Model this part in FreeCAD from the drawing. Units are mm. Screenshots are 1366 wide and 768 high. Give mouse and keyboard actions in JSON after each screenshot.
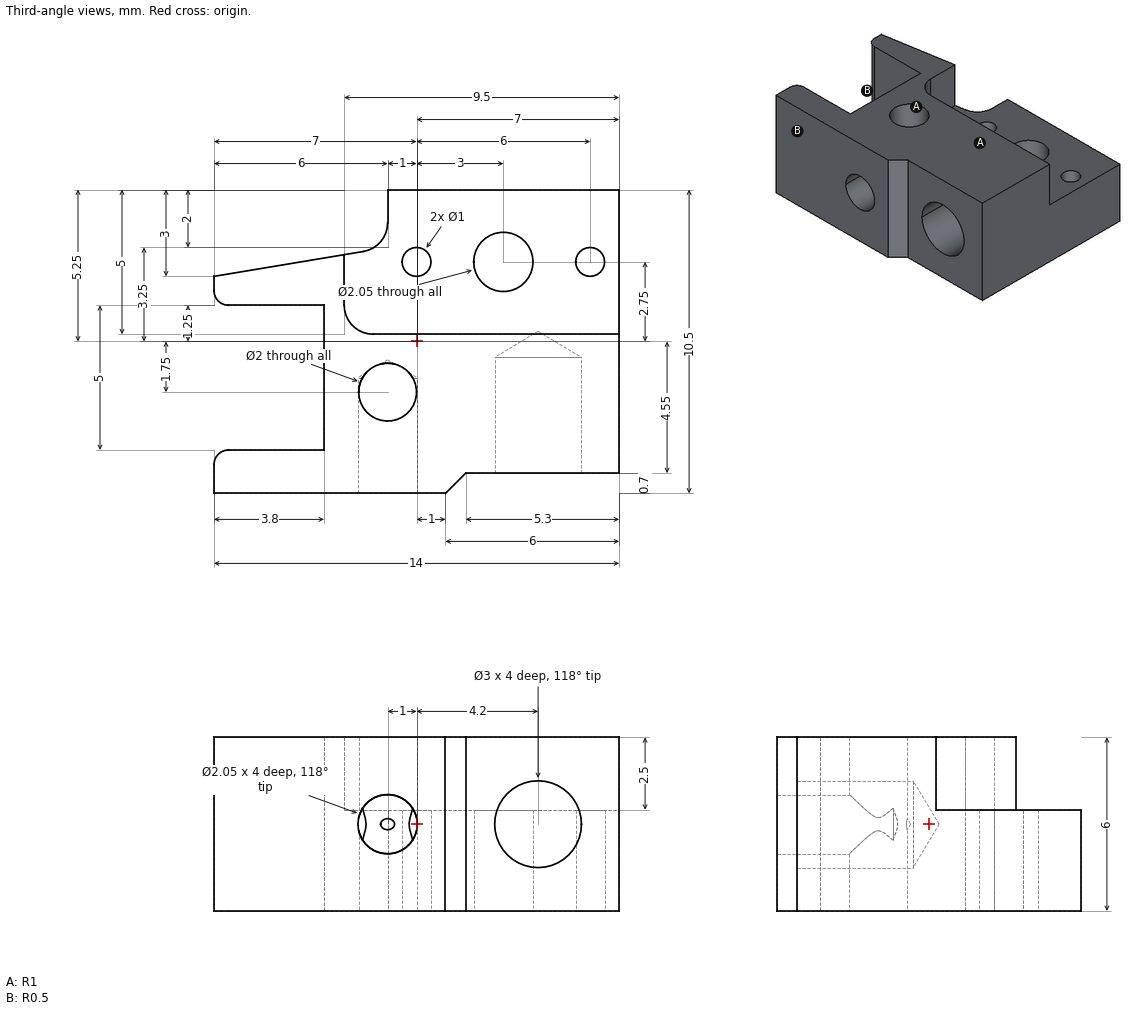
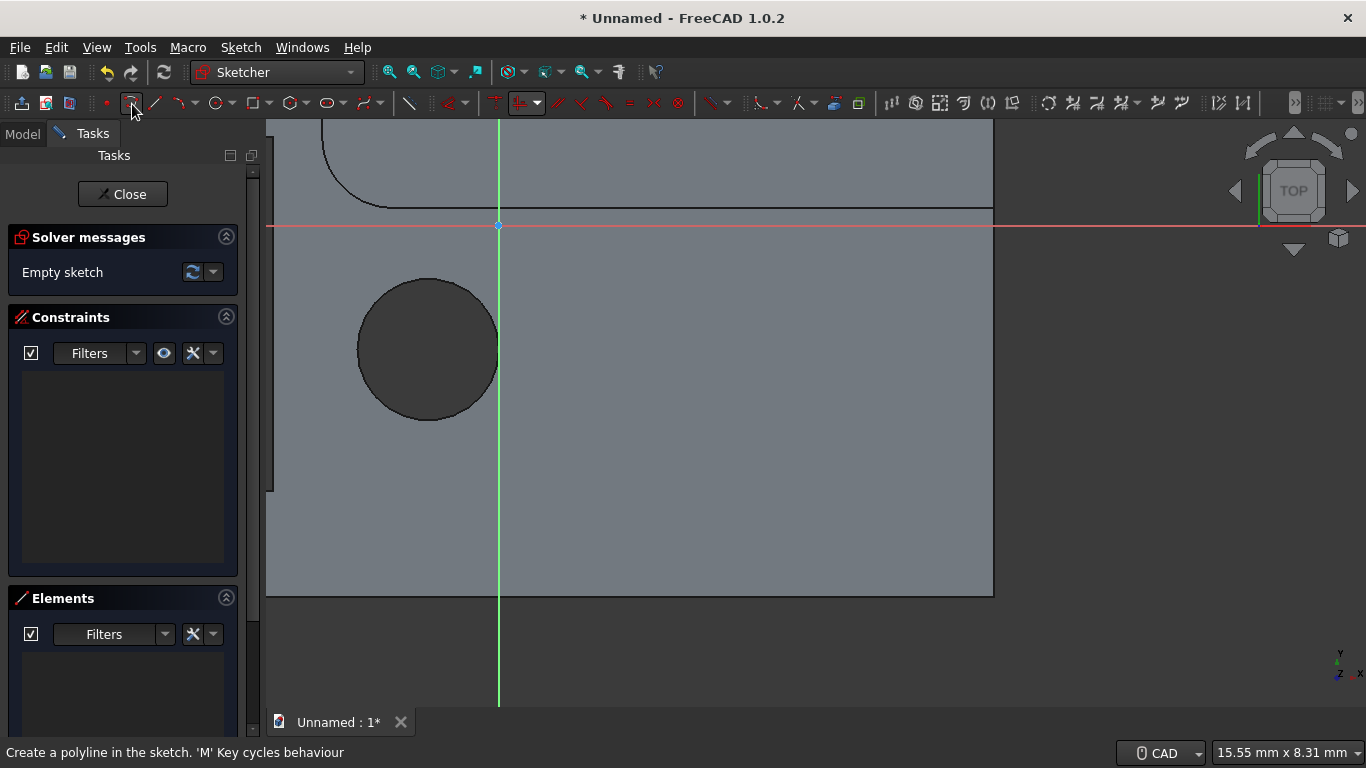
{"action": "left_click", "coordinate": [619, 548]}
{"action": "left_click", "coordinate": [570, 597]}
{"action": "left_click", "coordinate": [994, 597]}
{"action": "left_click", "coordinate": [994, 548]}
{"action": "left_click", "coordinate": [619, 549]}
{"action": "key", "text": "Escape"}
{"action": "key", "text": "Escape"}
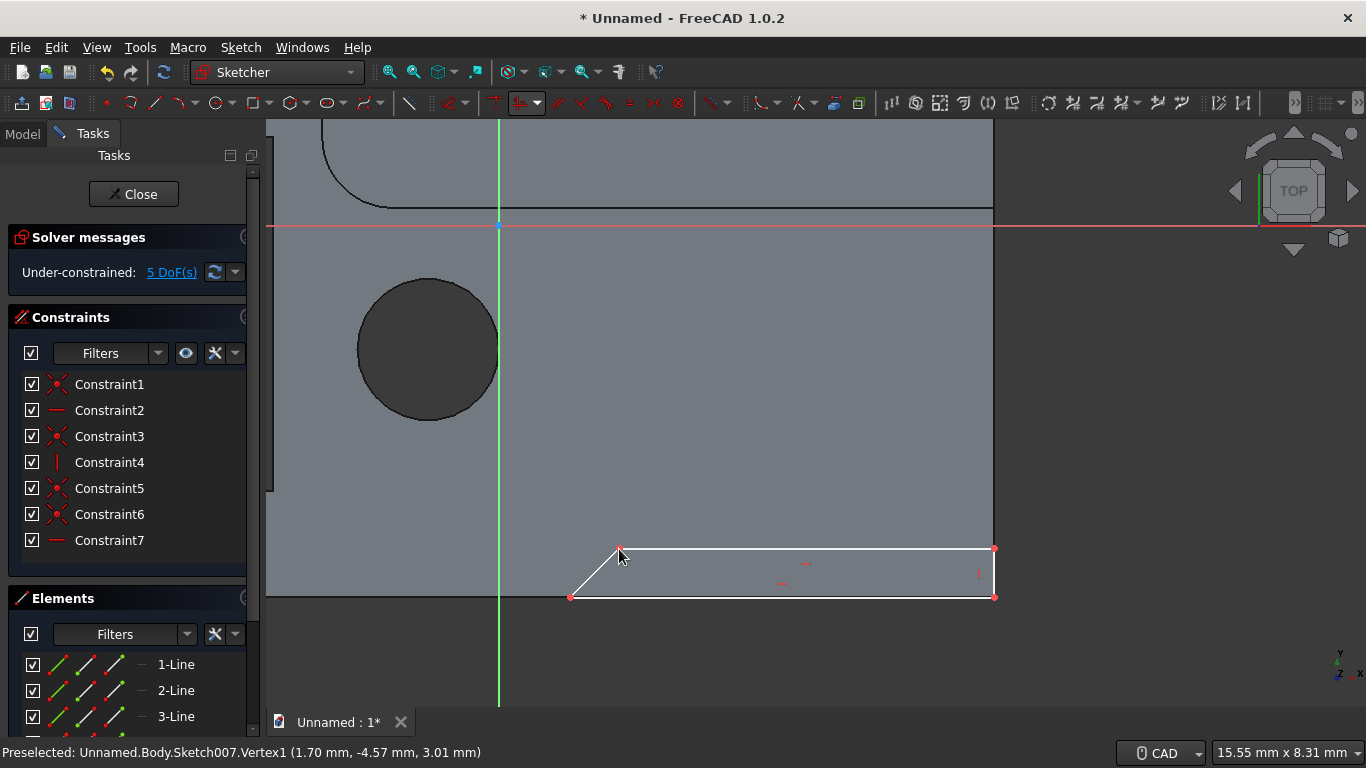
{"action": "left_click", "coordinate": [448, 104]}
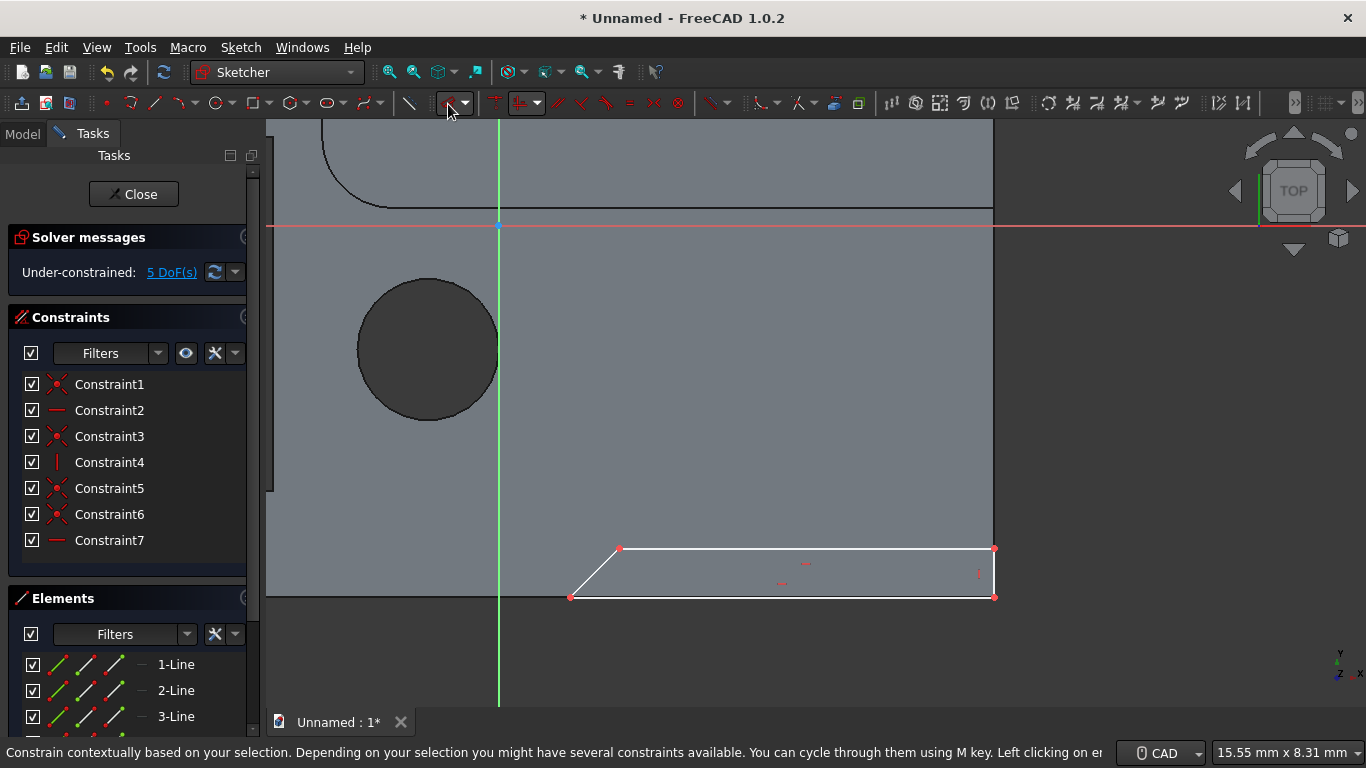
{"action": "left_click", "coordinate": [697, 598]}
{"action": "left_click", "coordinate": [782, 632]}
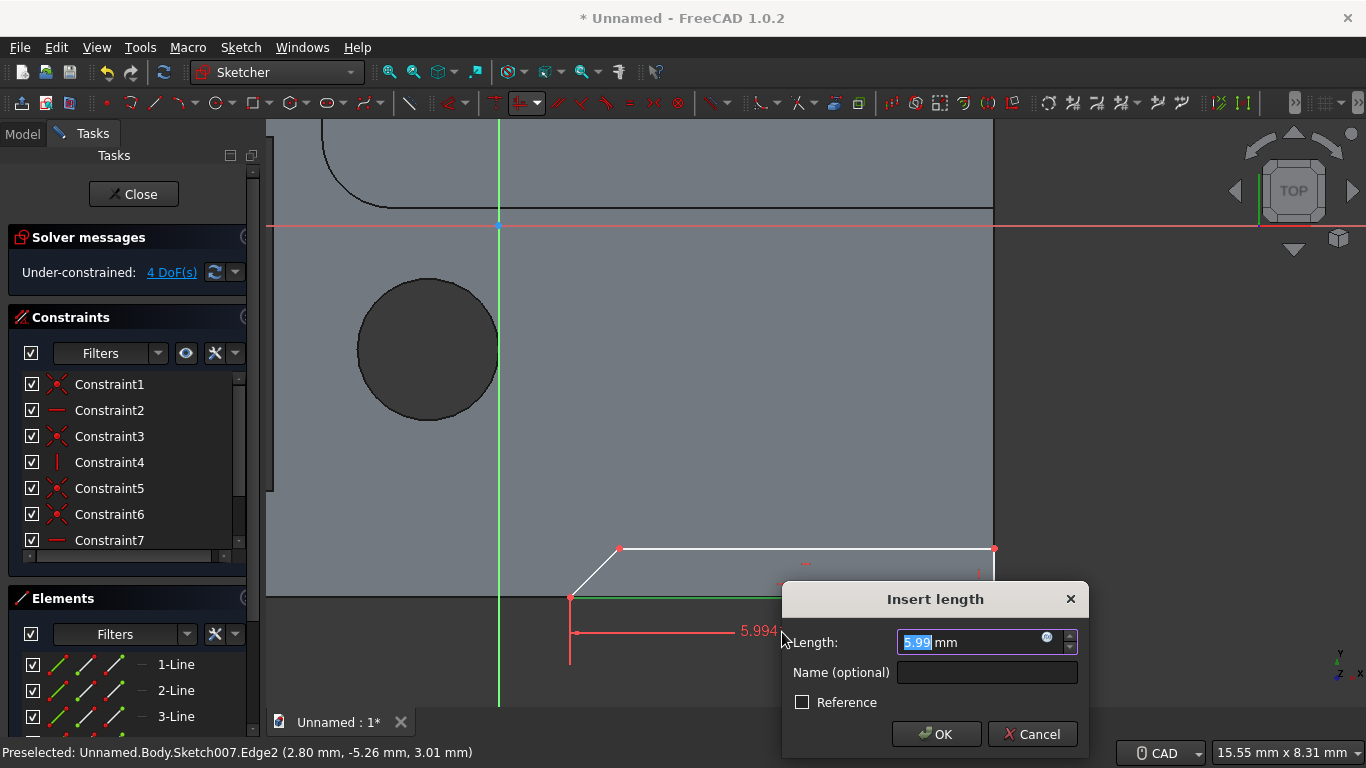
{"action": "type", "text": "6"}
{"action": "key", "text": "Return"}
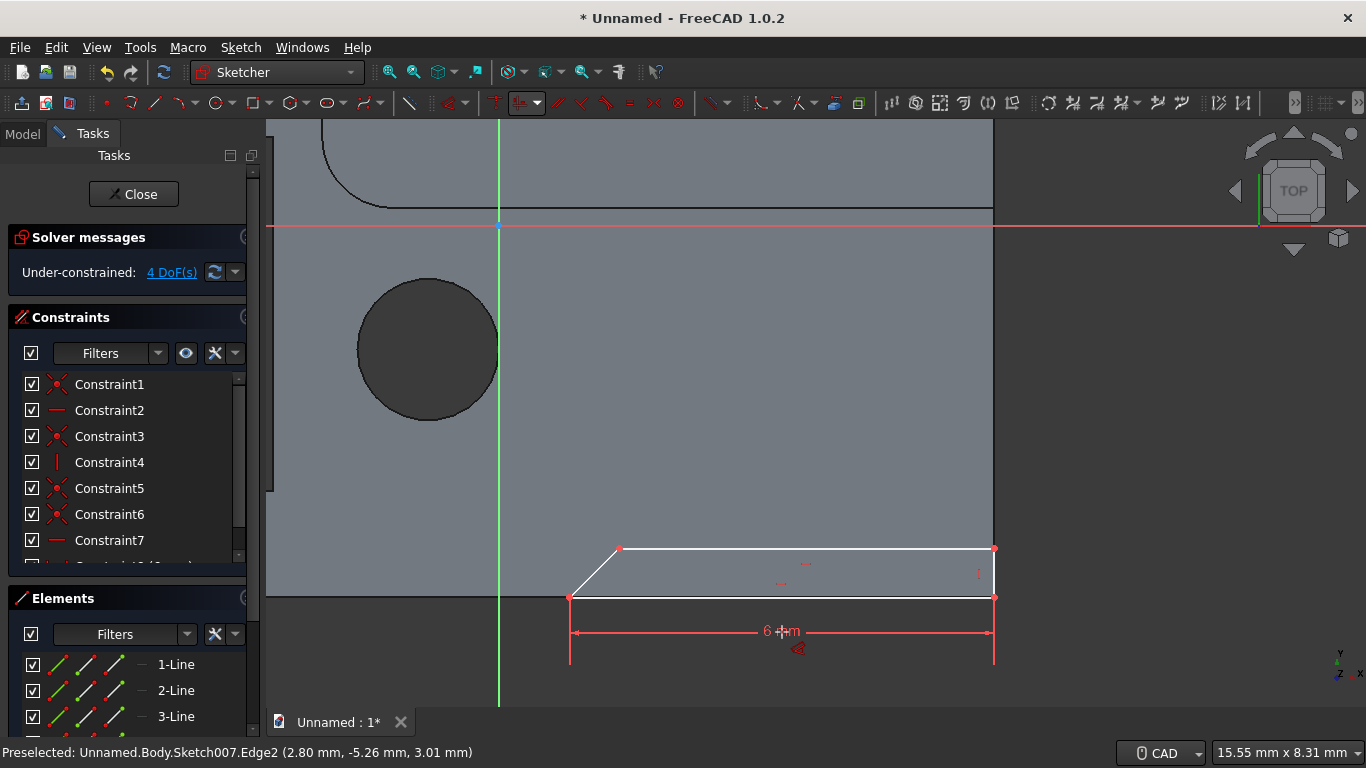
{"action": "left_click", "coordinate": [570, 598]}
{"action": "left_click", "coordinate": [534, 632]}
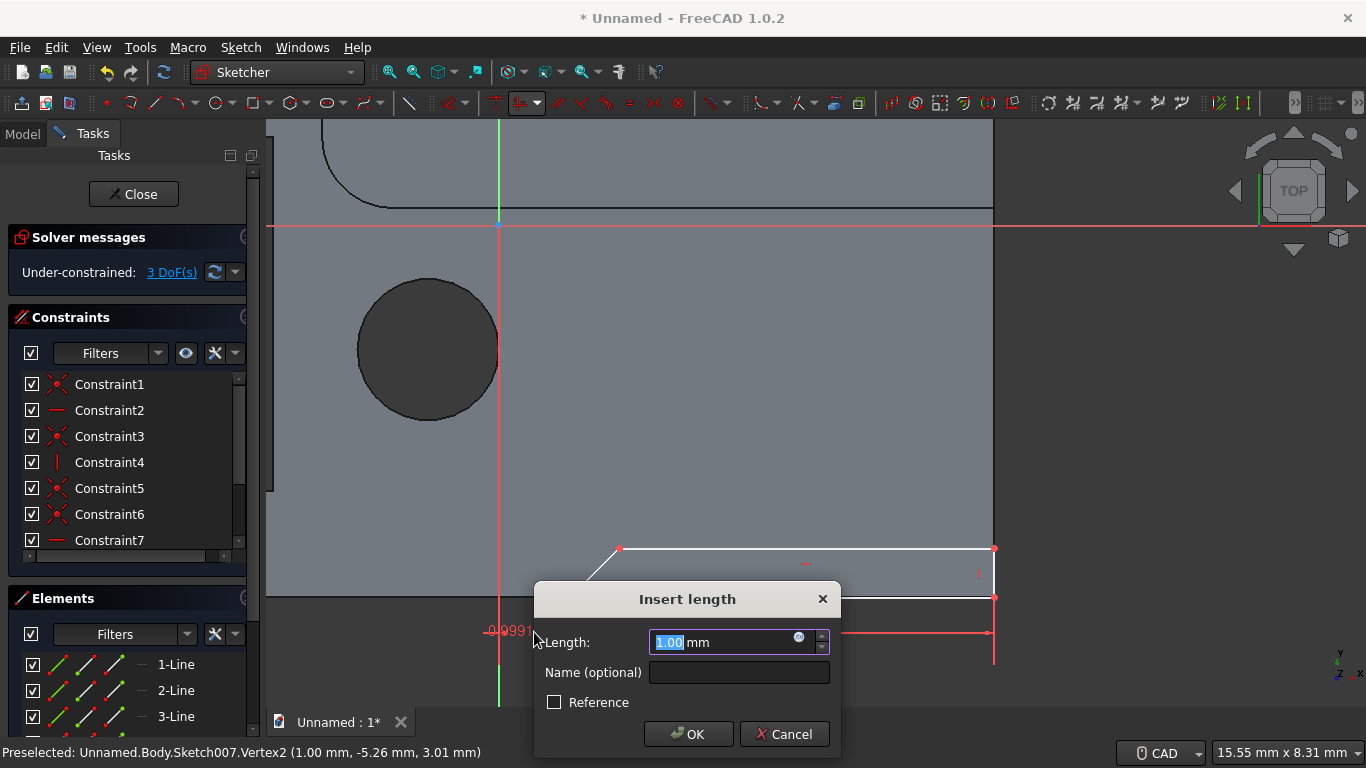
{"action": "type", "text": "1"}
{"action": "key", "text": "Return"}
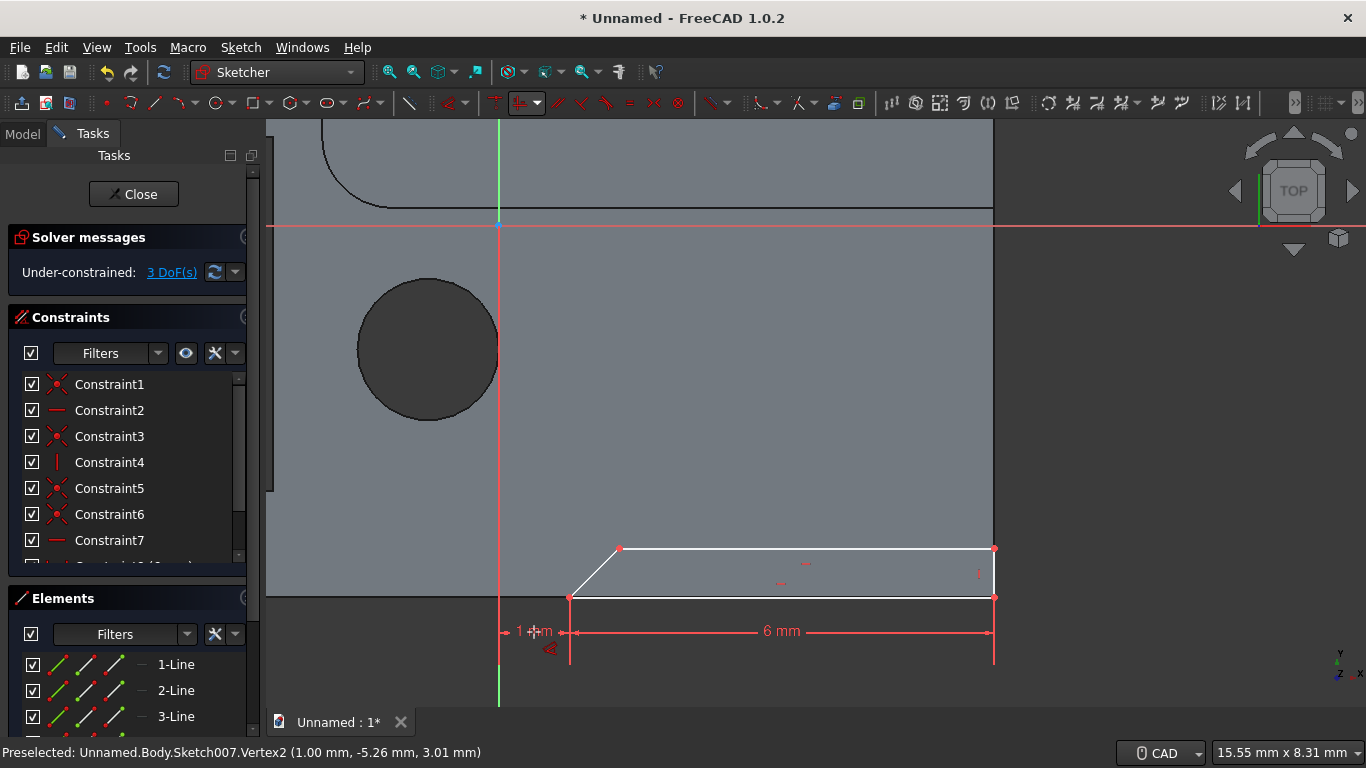
{"action": "left_click", "coordinate": [994, 583]}
{"action": "left_click", "coordinate": [1028, 574]}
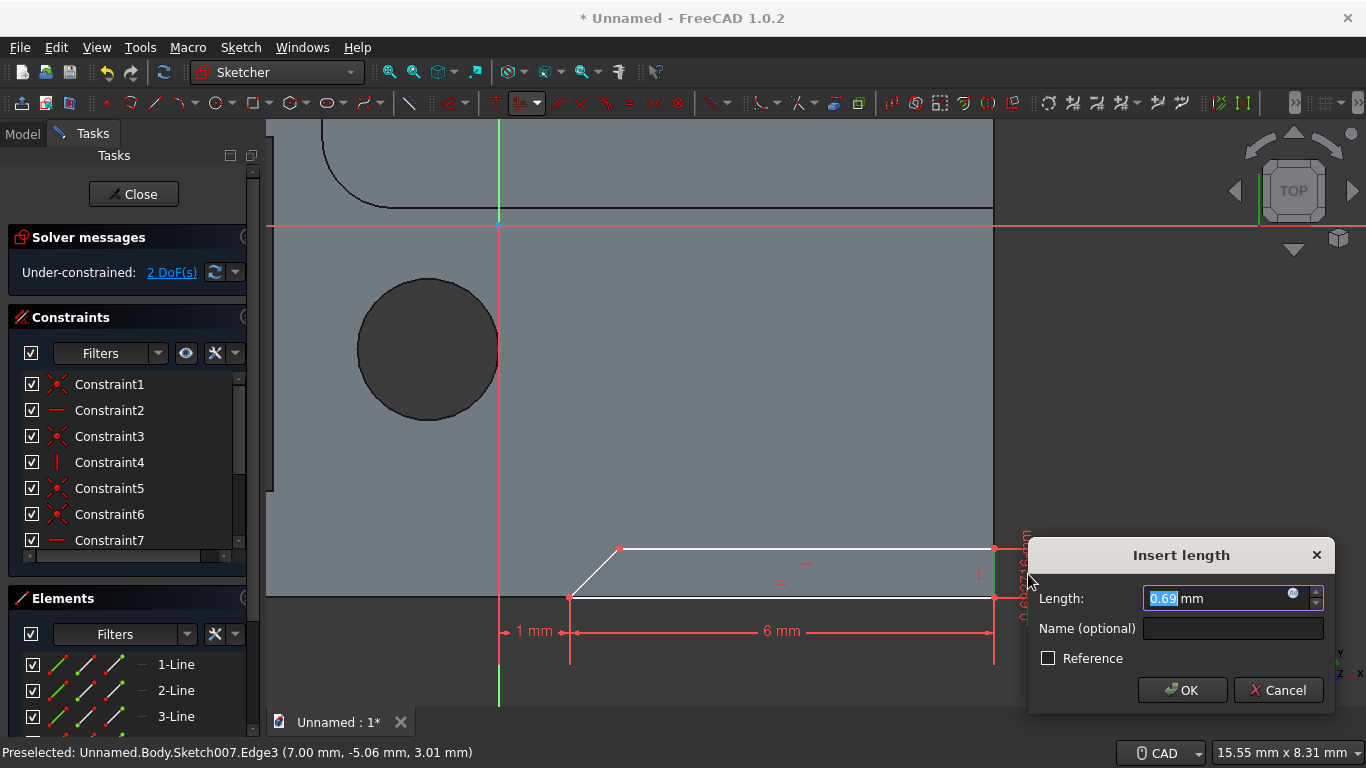
{"action": "type", "text": "0.7"}
{"action": "key", "text": "Return"}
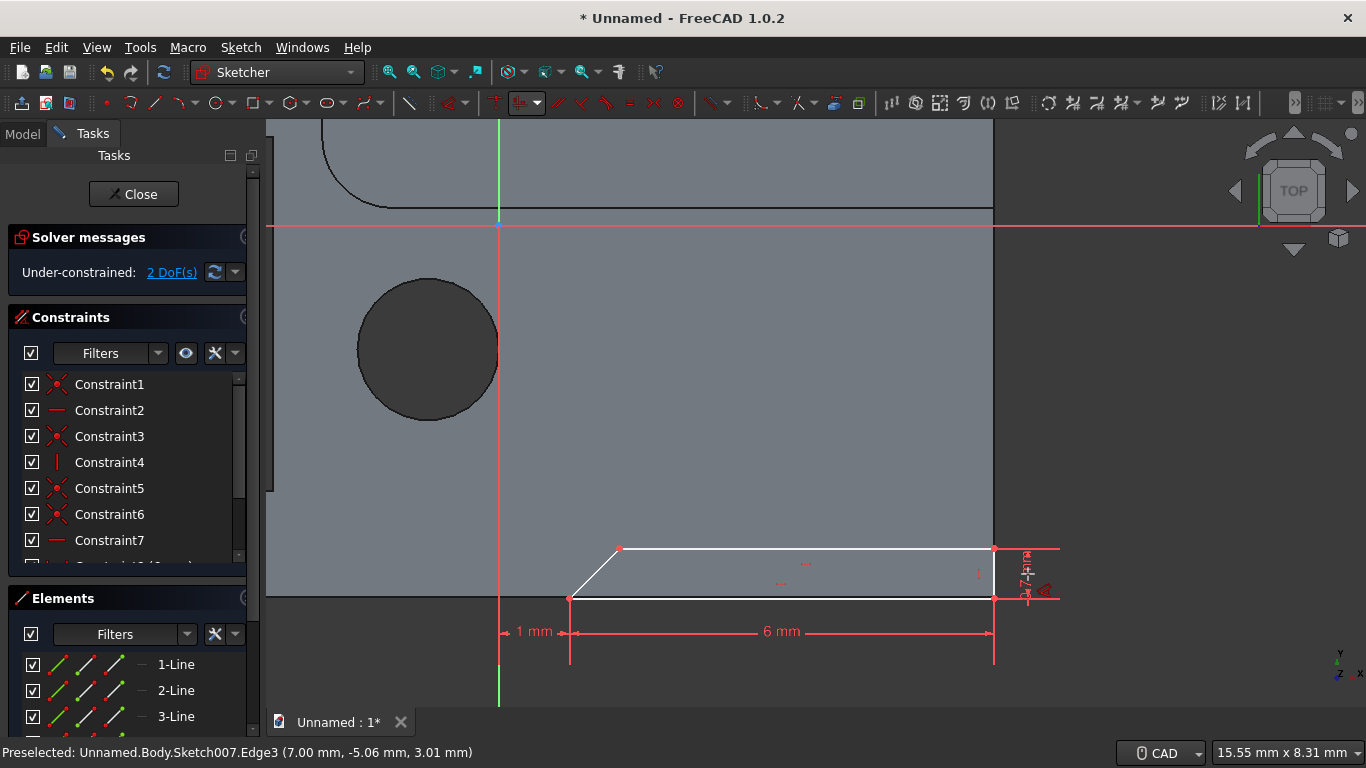
{"action": "left_click", "coordinate": [882, 549]}
{"action": "left_click", "coordinate": [807, 583]}